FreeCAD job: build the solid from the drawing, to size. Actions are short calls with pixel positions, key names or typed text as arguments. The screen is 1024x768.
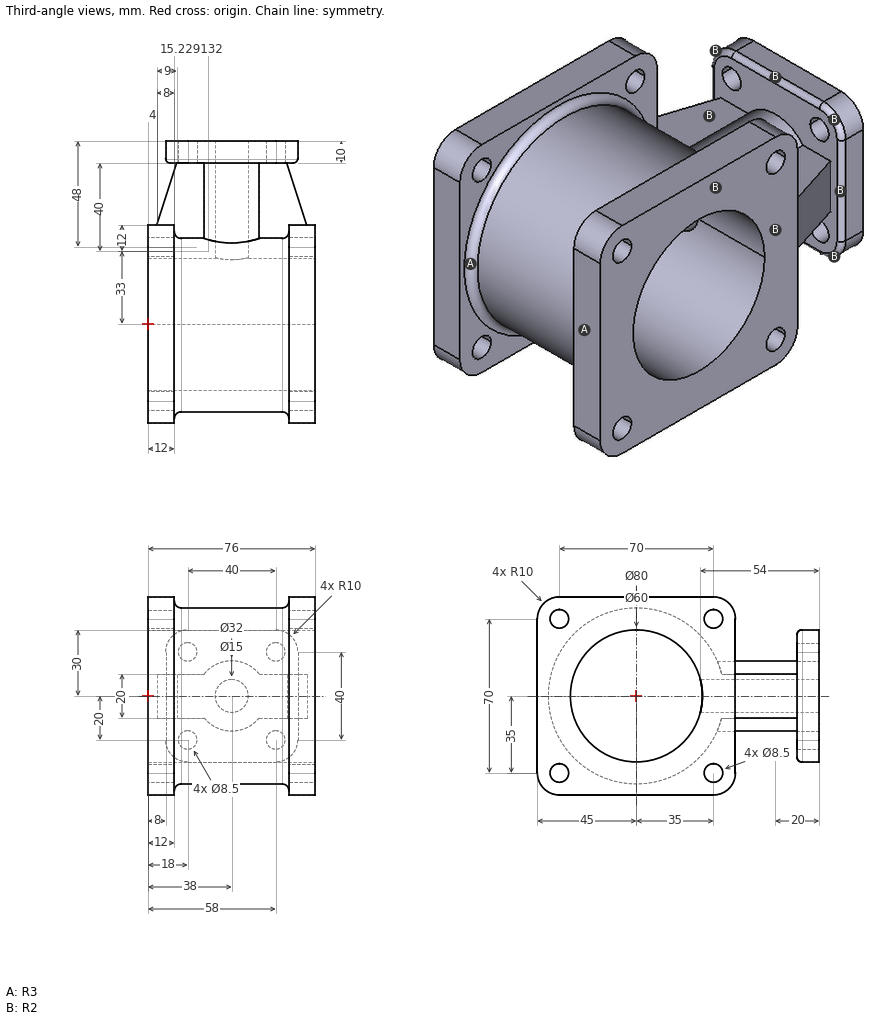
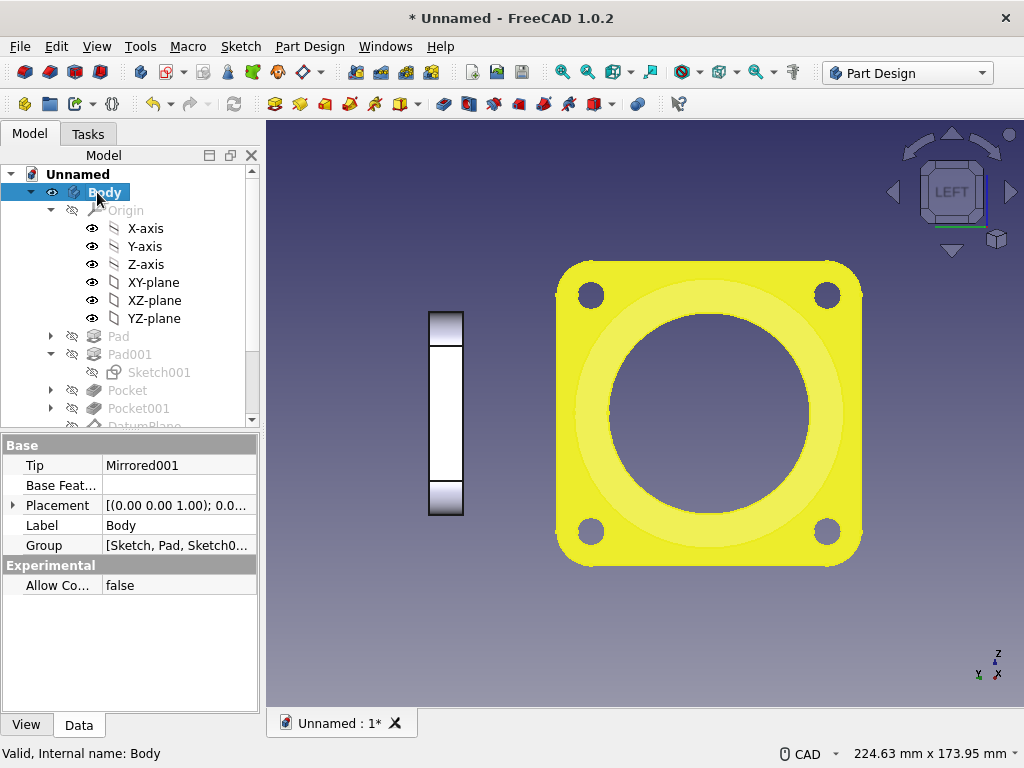
click(148, 585)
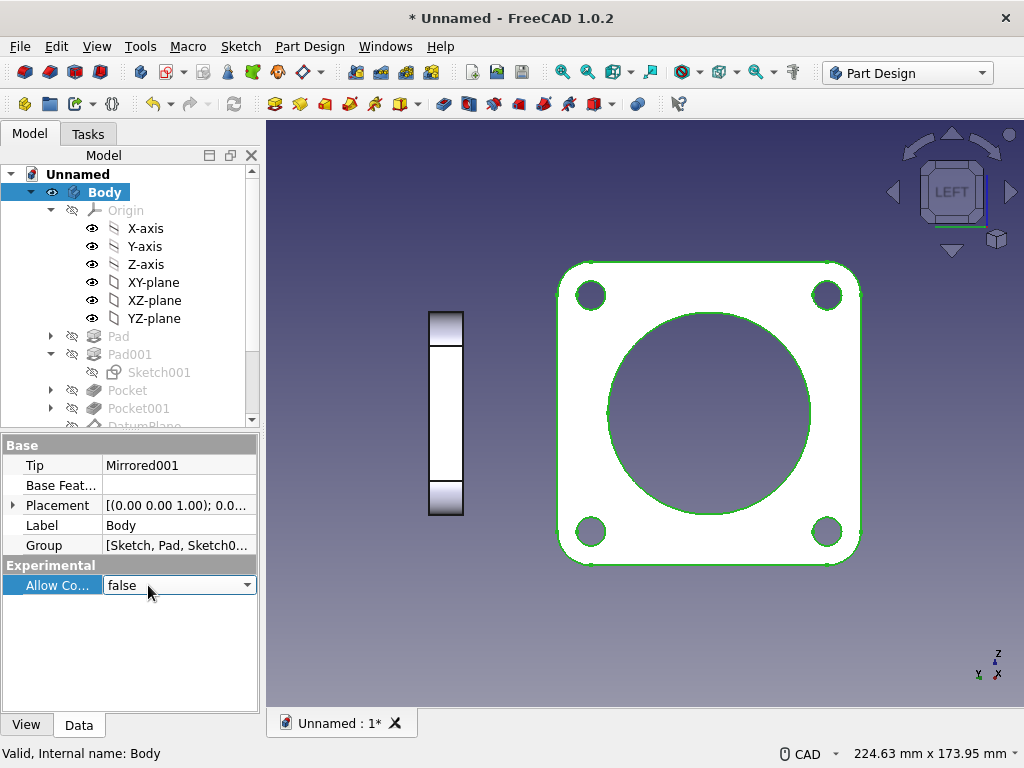
click(148, 585)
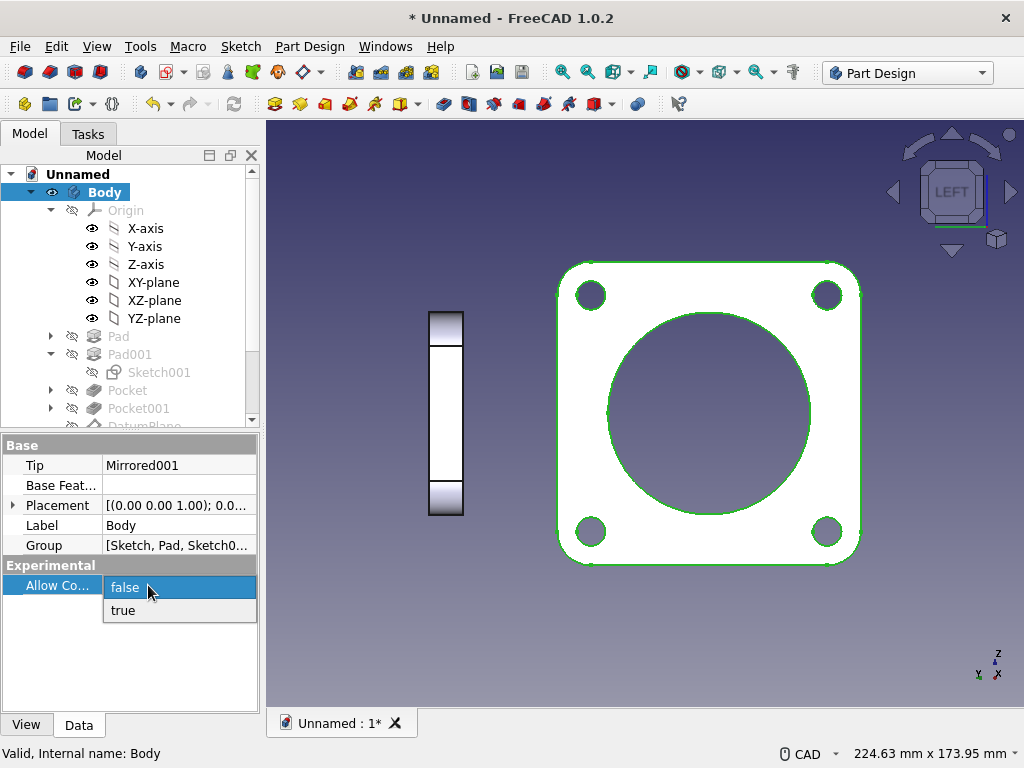
click(178, 610)
key(Return)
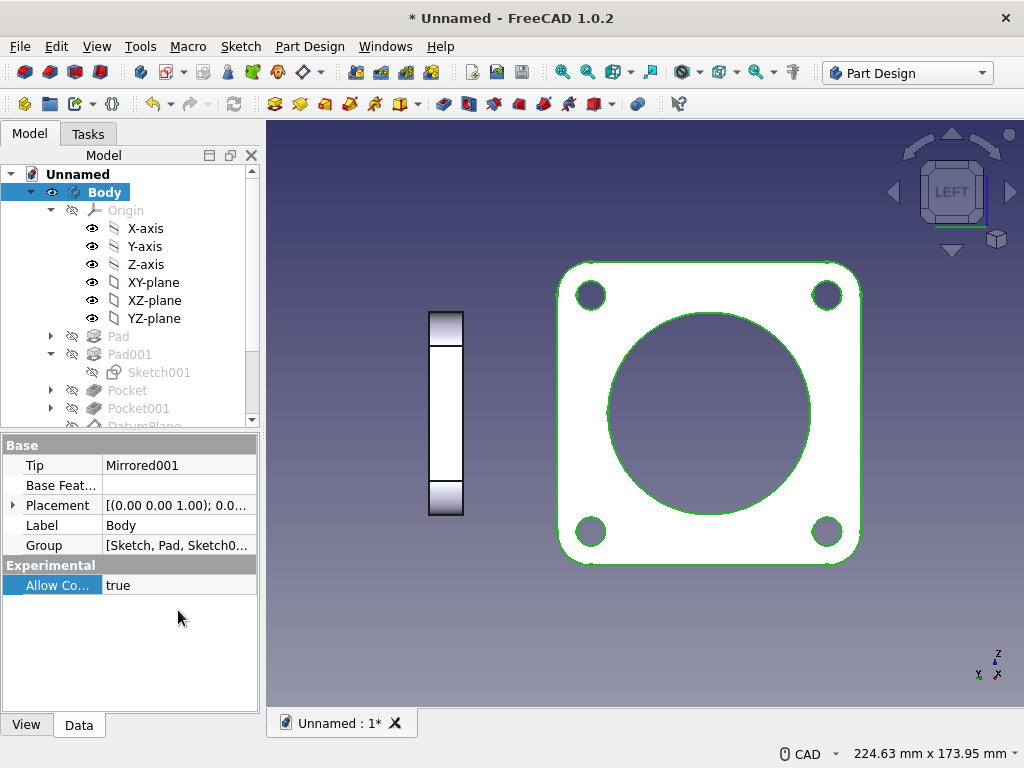
scroll(101, 296, down, 3)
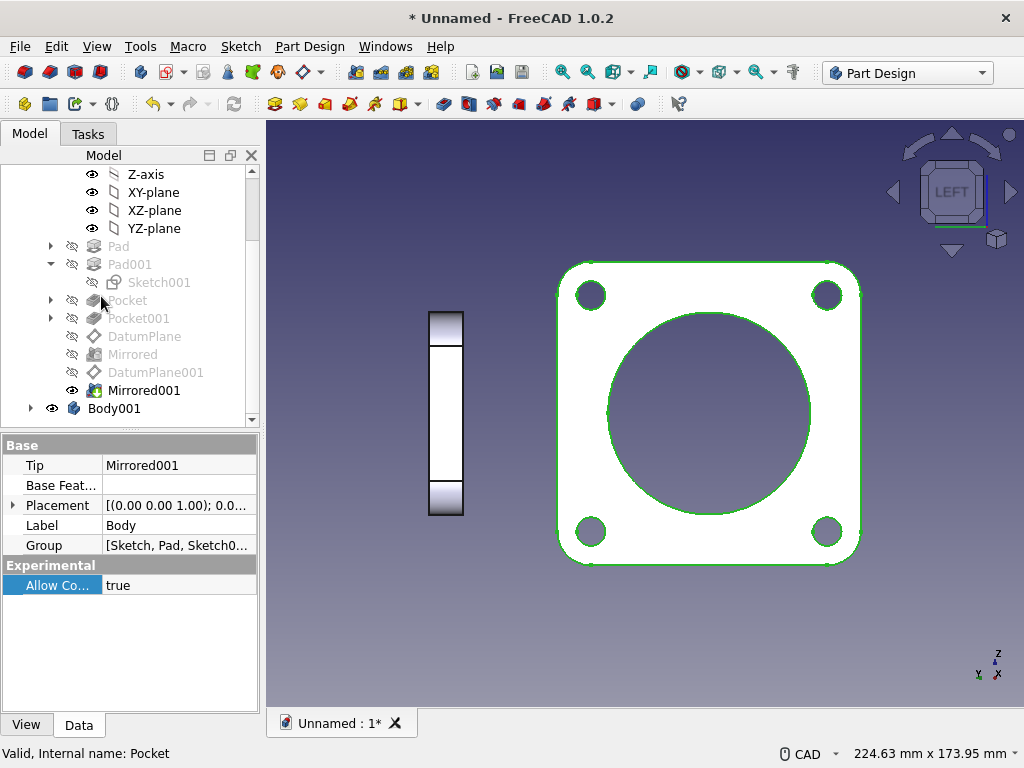
click(97, 408)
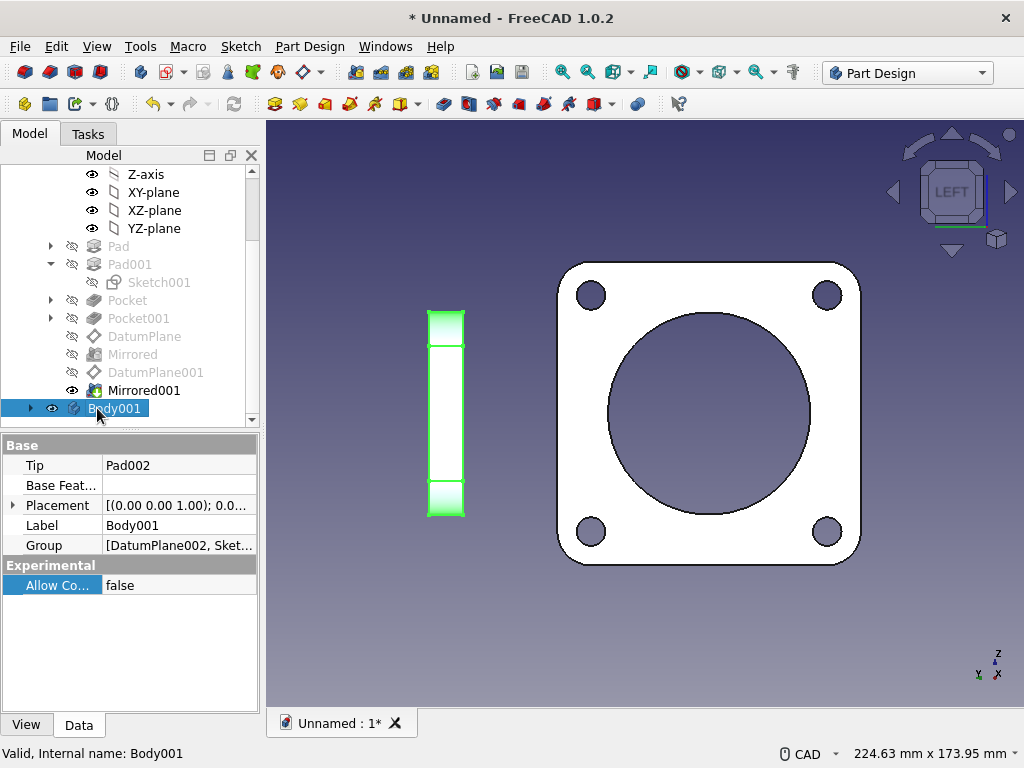
click(638, 104)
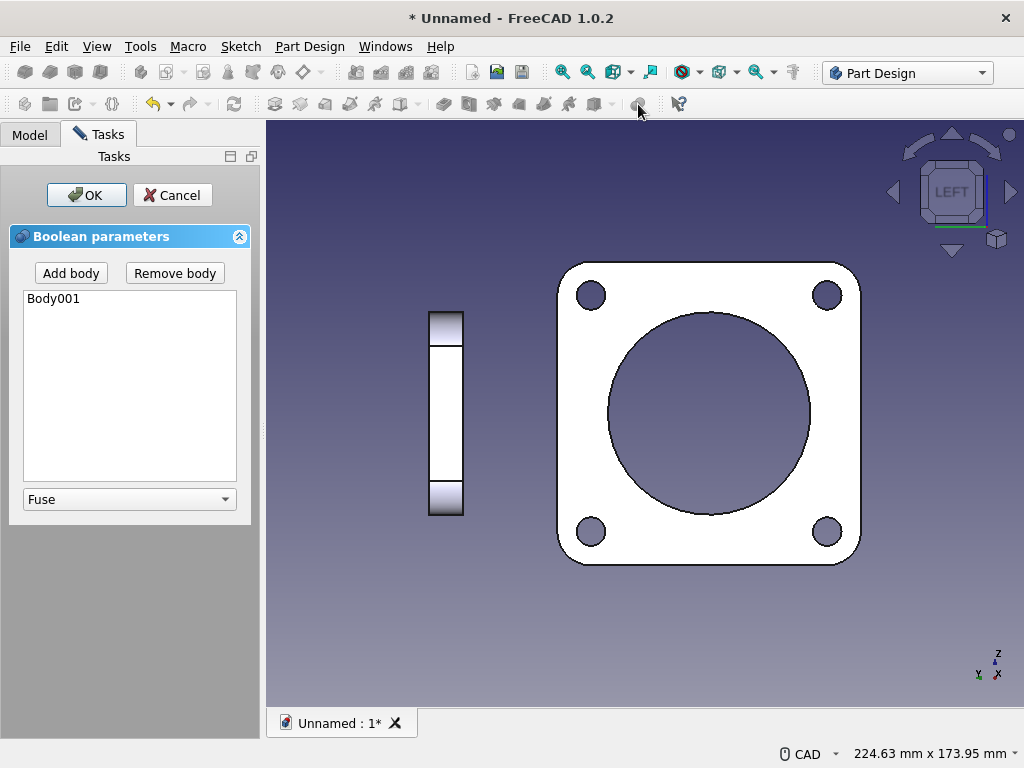
click(87, 195)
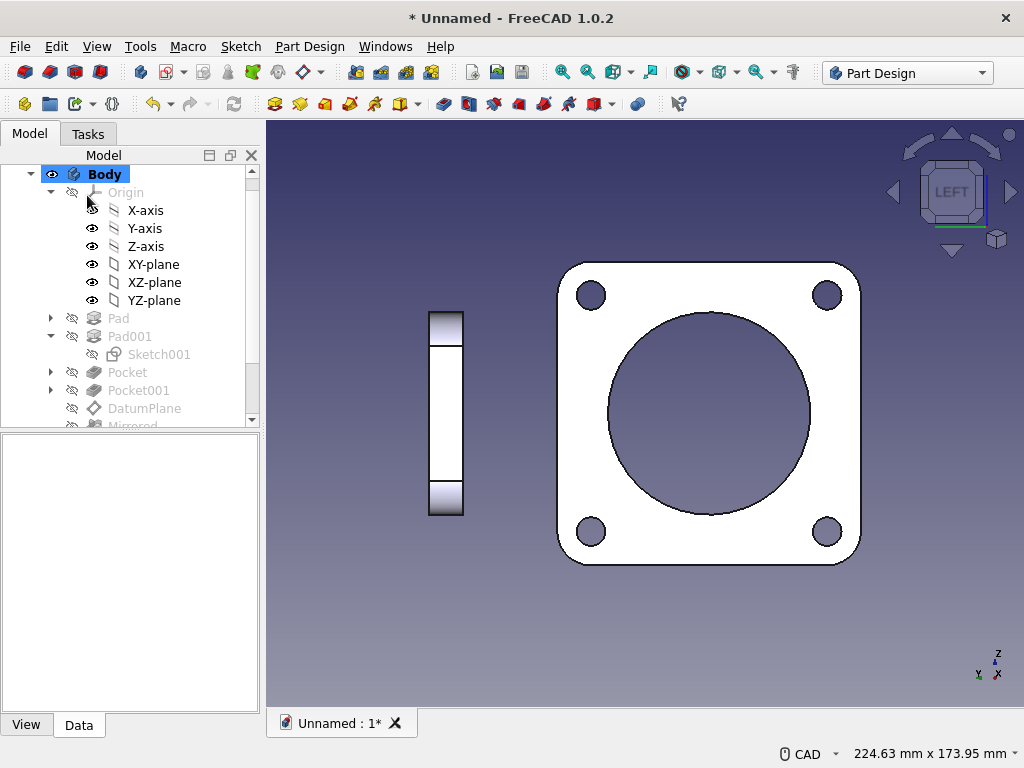
key(4)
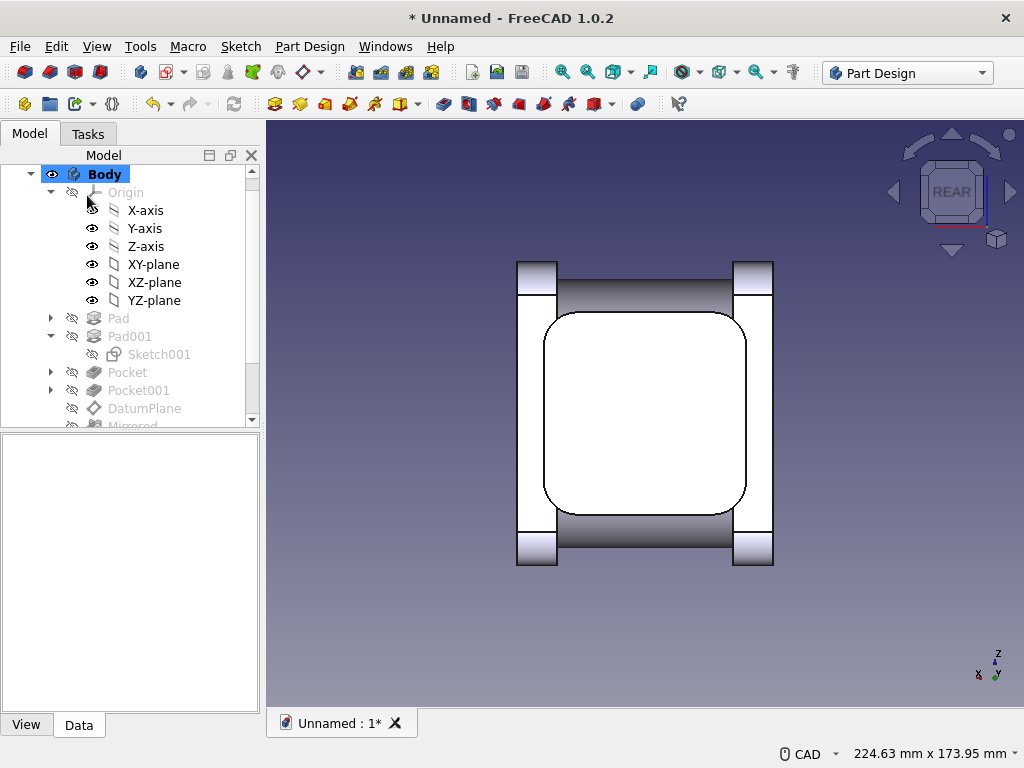
click(645, 412)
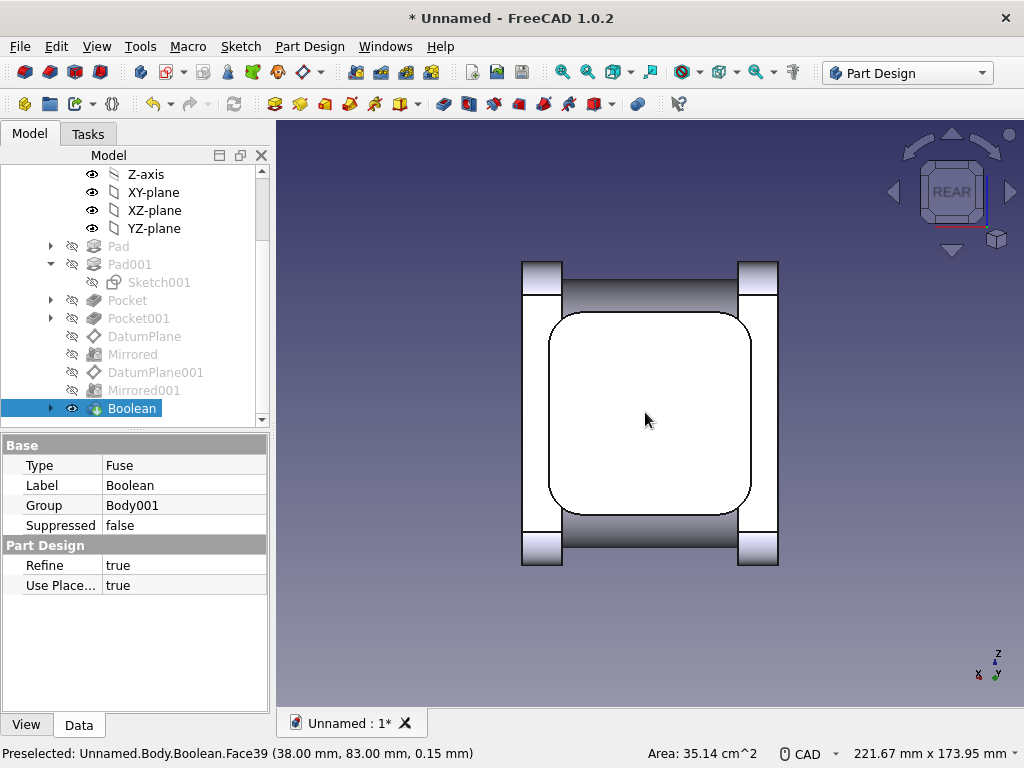
click(166, 72)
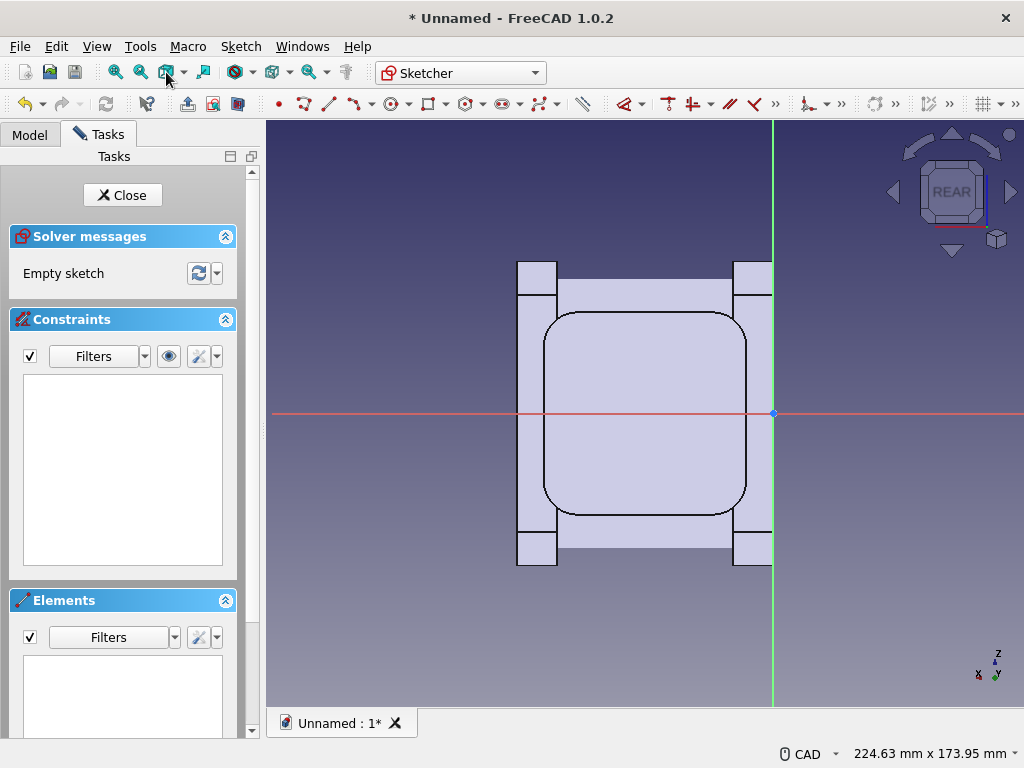
scroll(768, 413, up, 4)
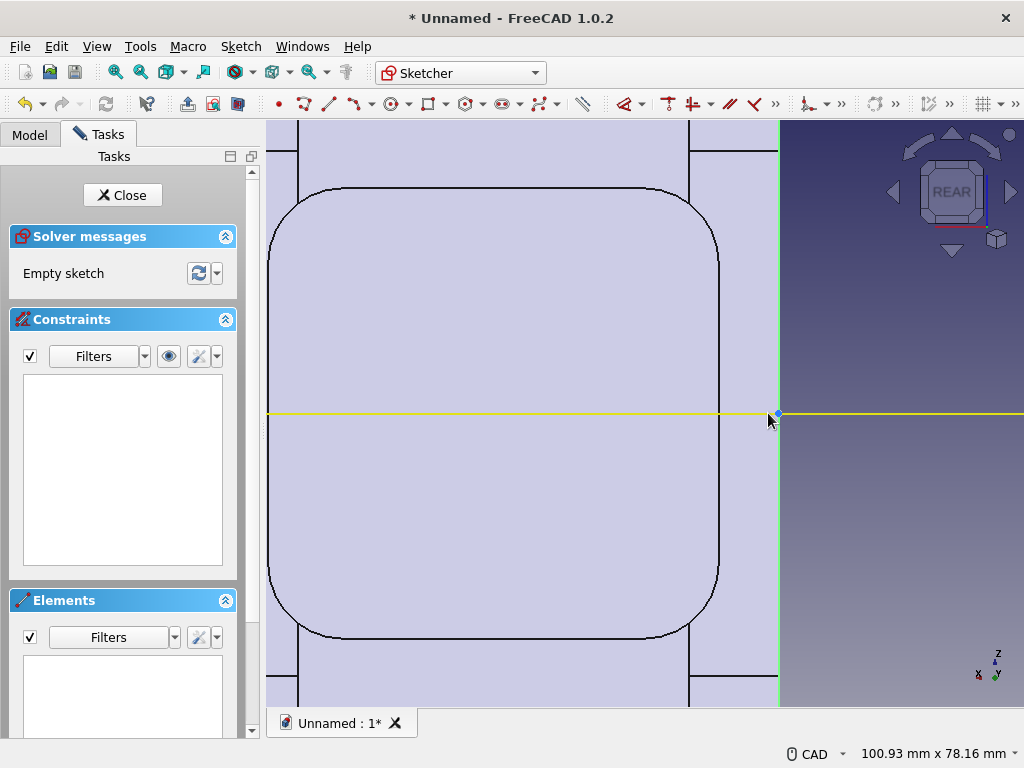
click(390, 104)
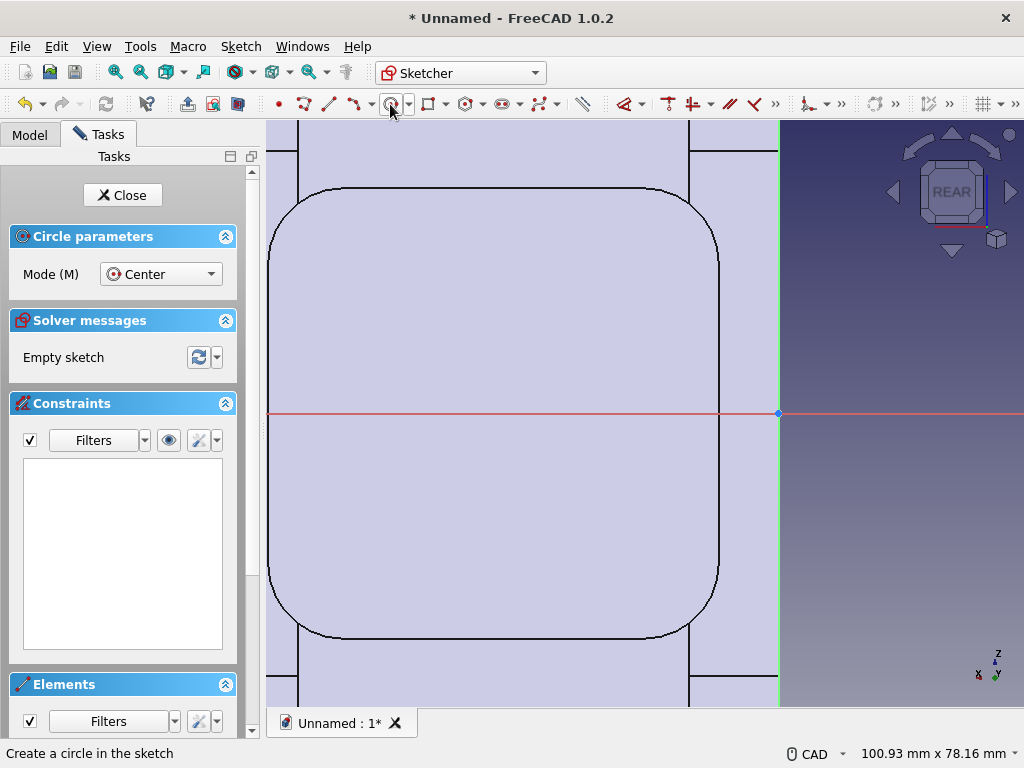
click(493, 413)
click(578, 329)
key(Escape)